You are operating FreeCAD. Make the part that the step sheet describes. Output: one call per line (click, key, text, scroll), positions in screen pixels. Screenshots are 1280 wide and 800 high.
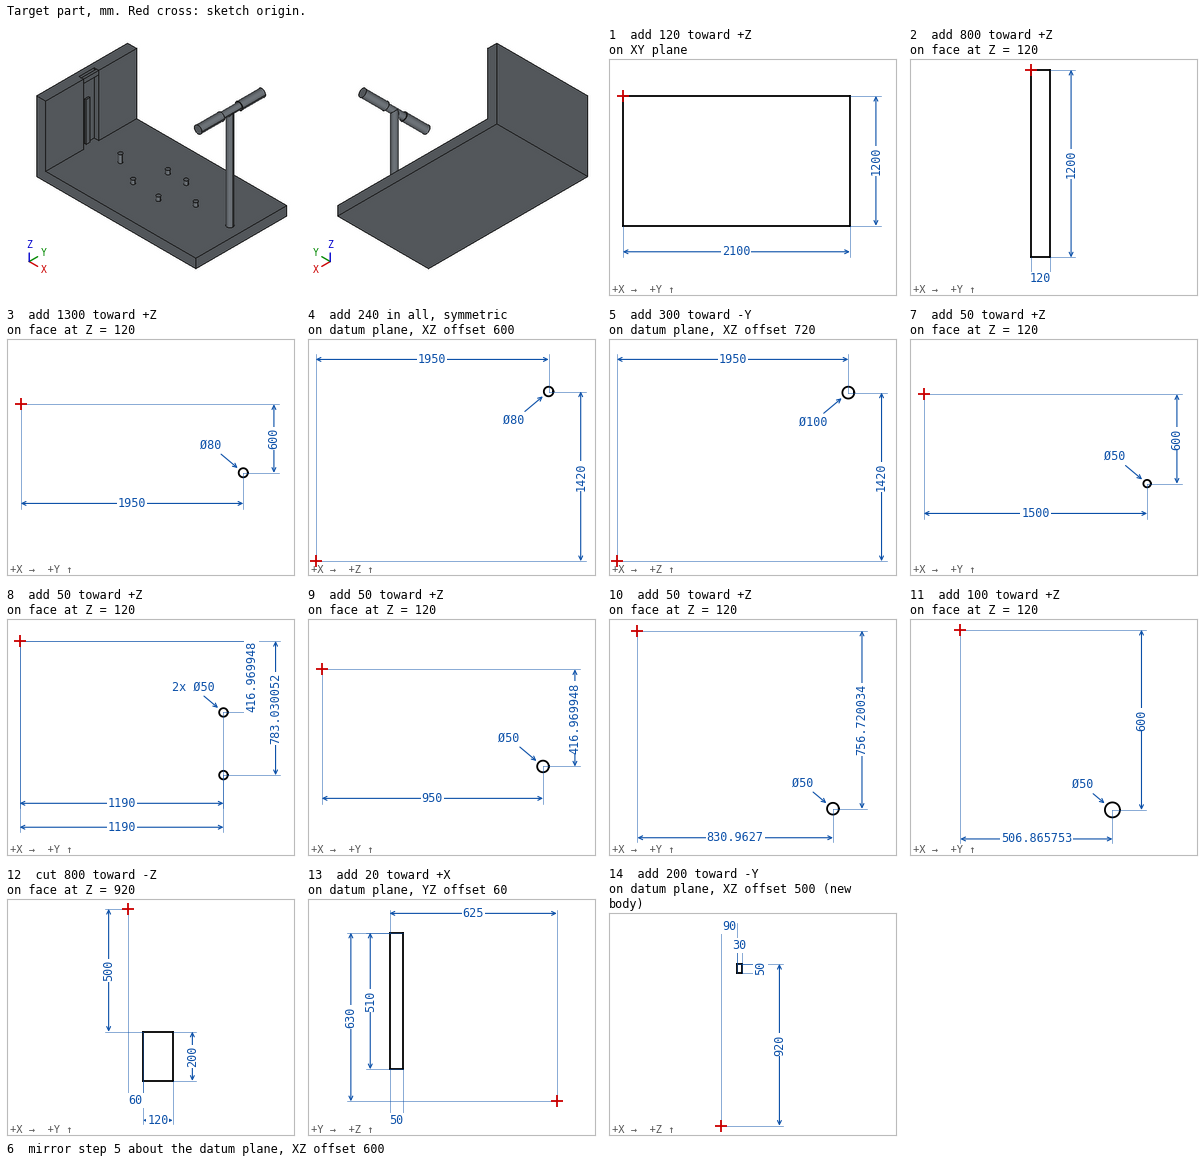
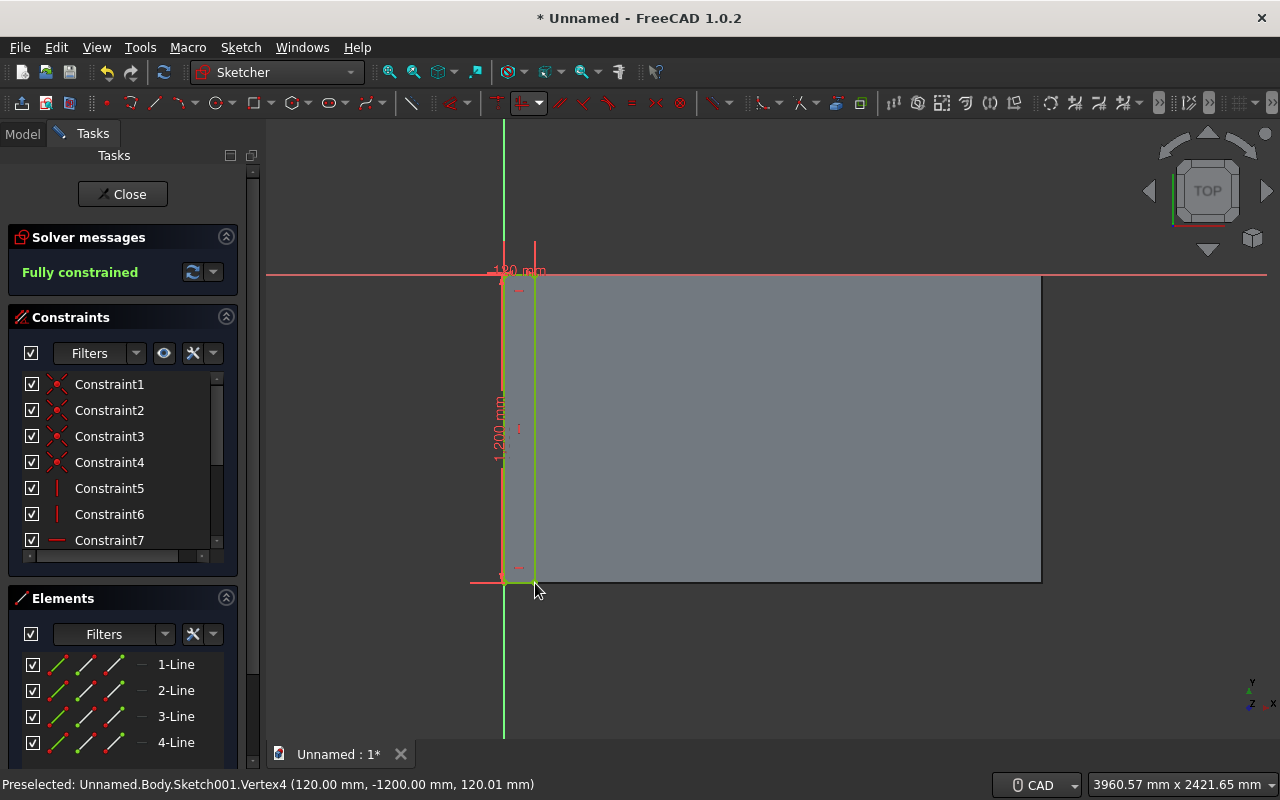
click(123, 194)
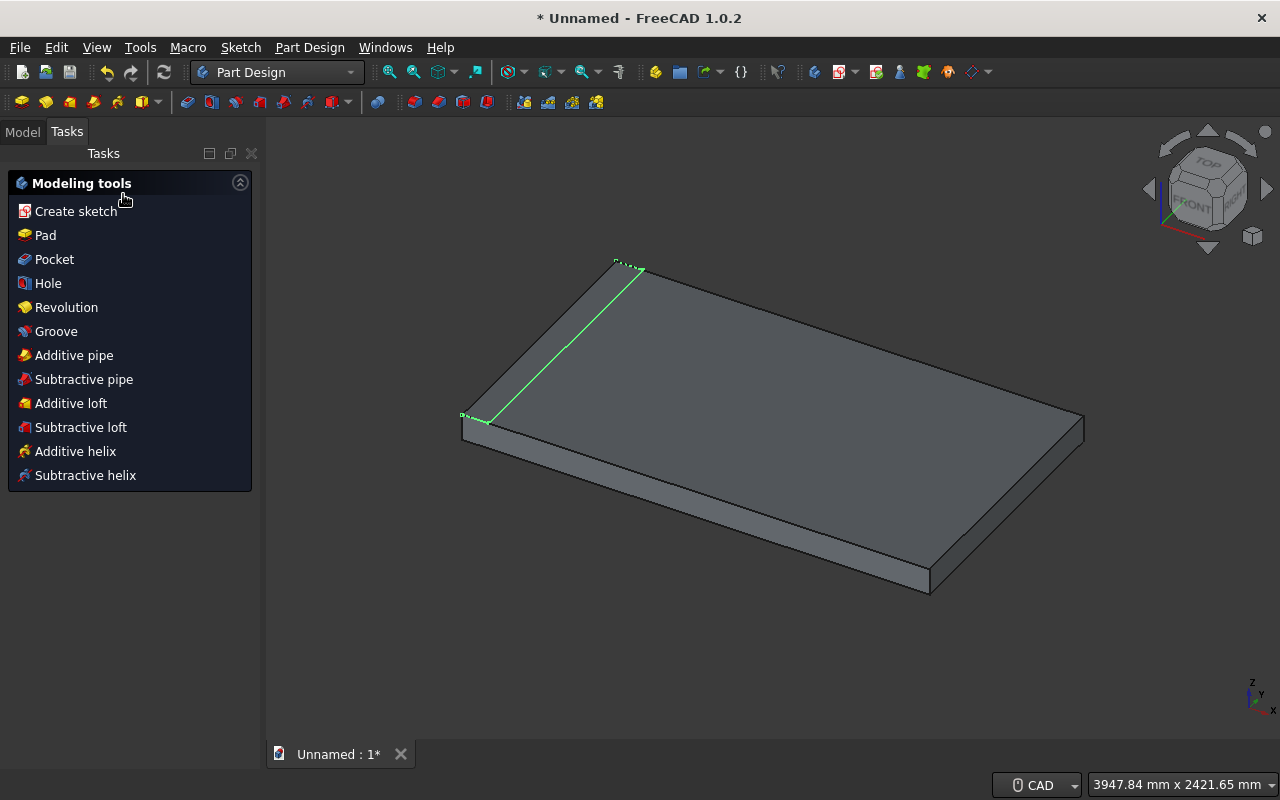
click(22, 102)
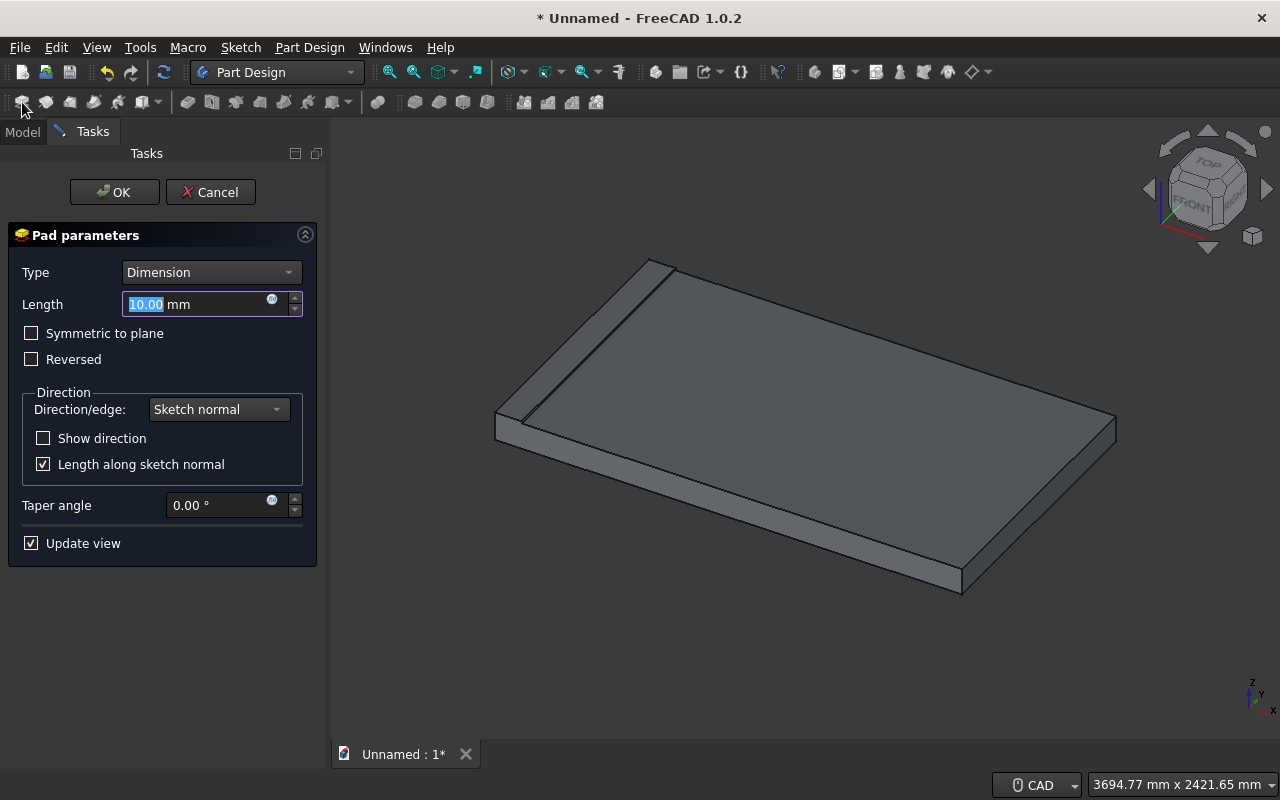
text(800)
key(Tab)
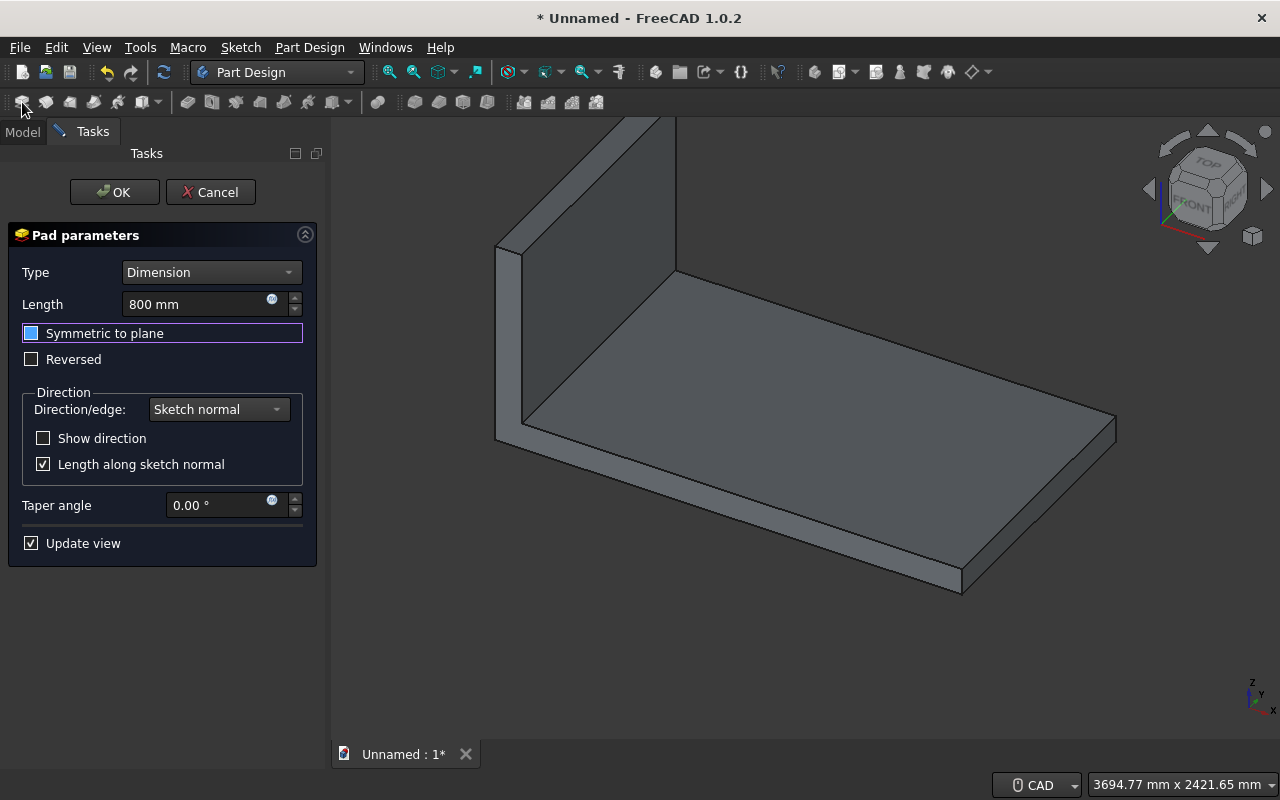
click(115, 192)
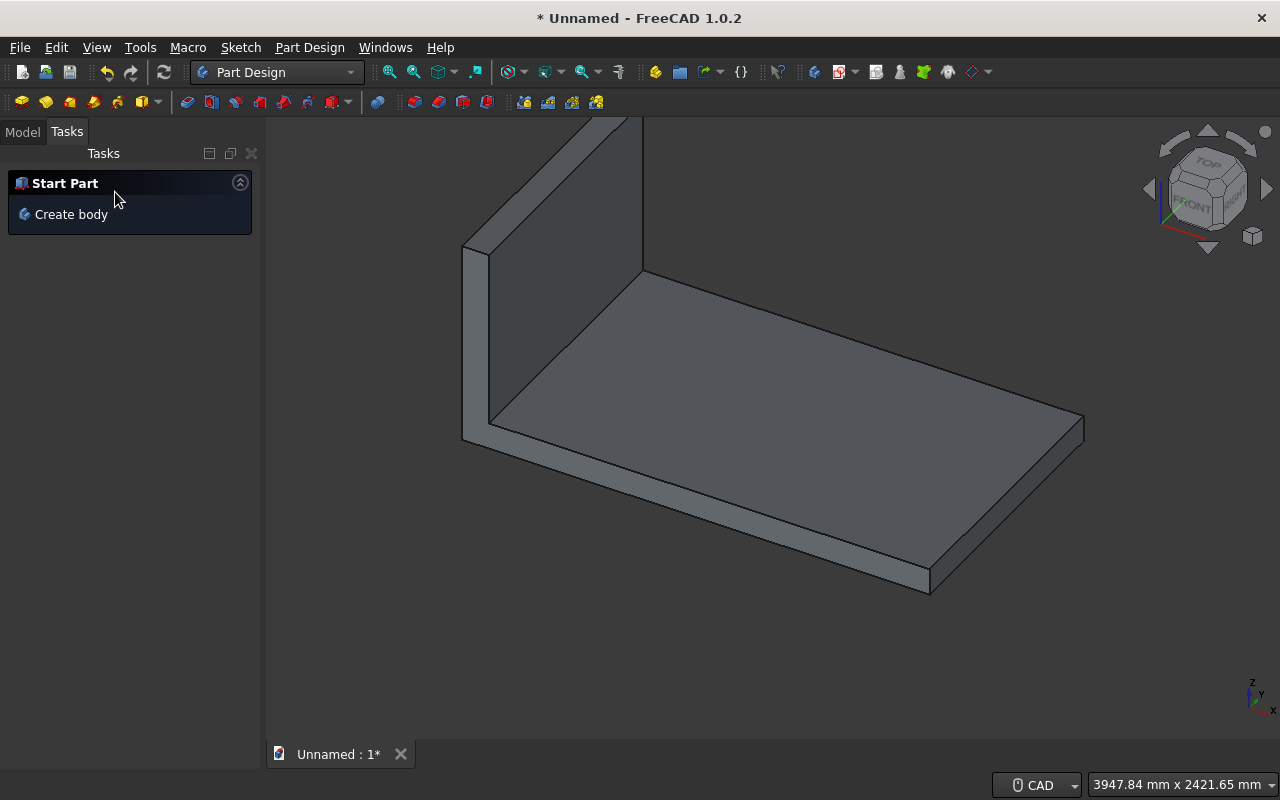
key(v)
key(f)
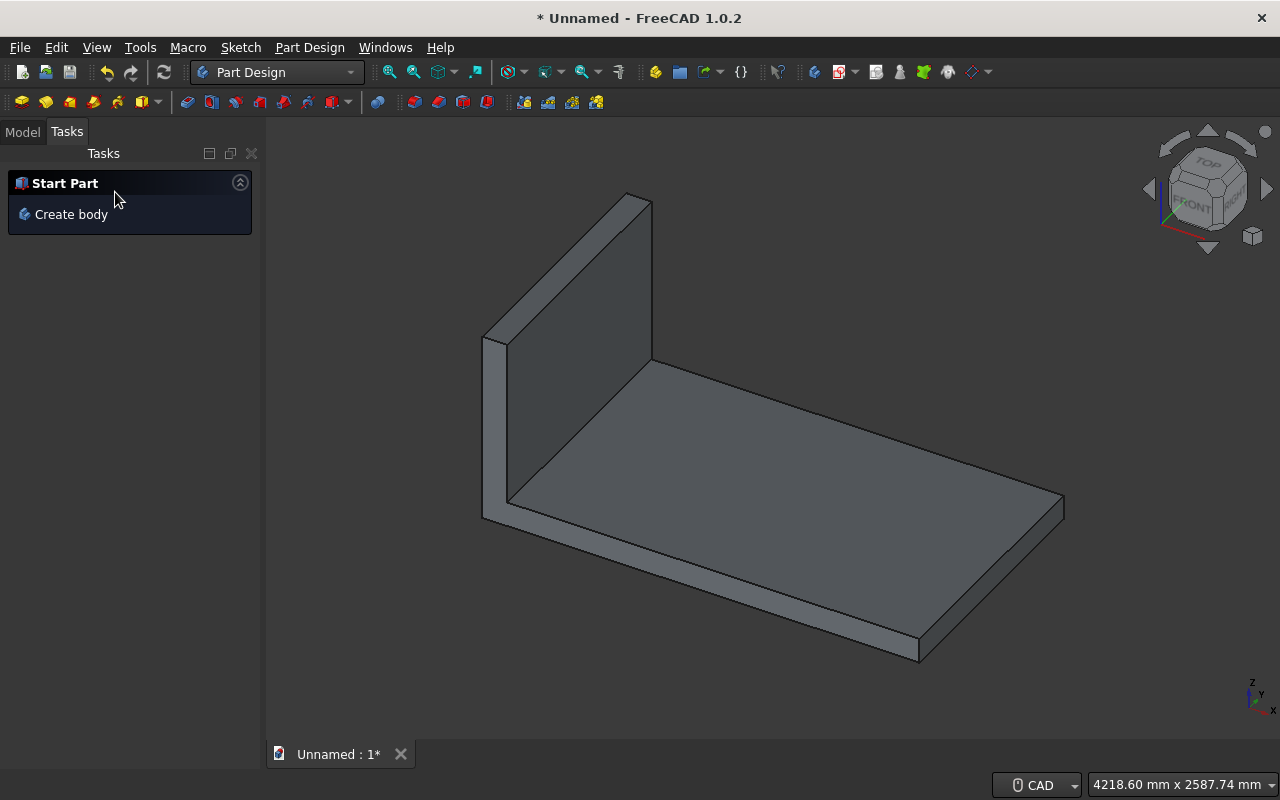
click(844, 518)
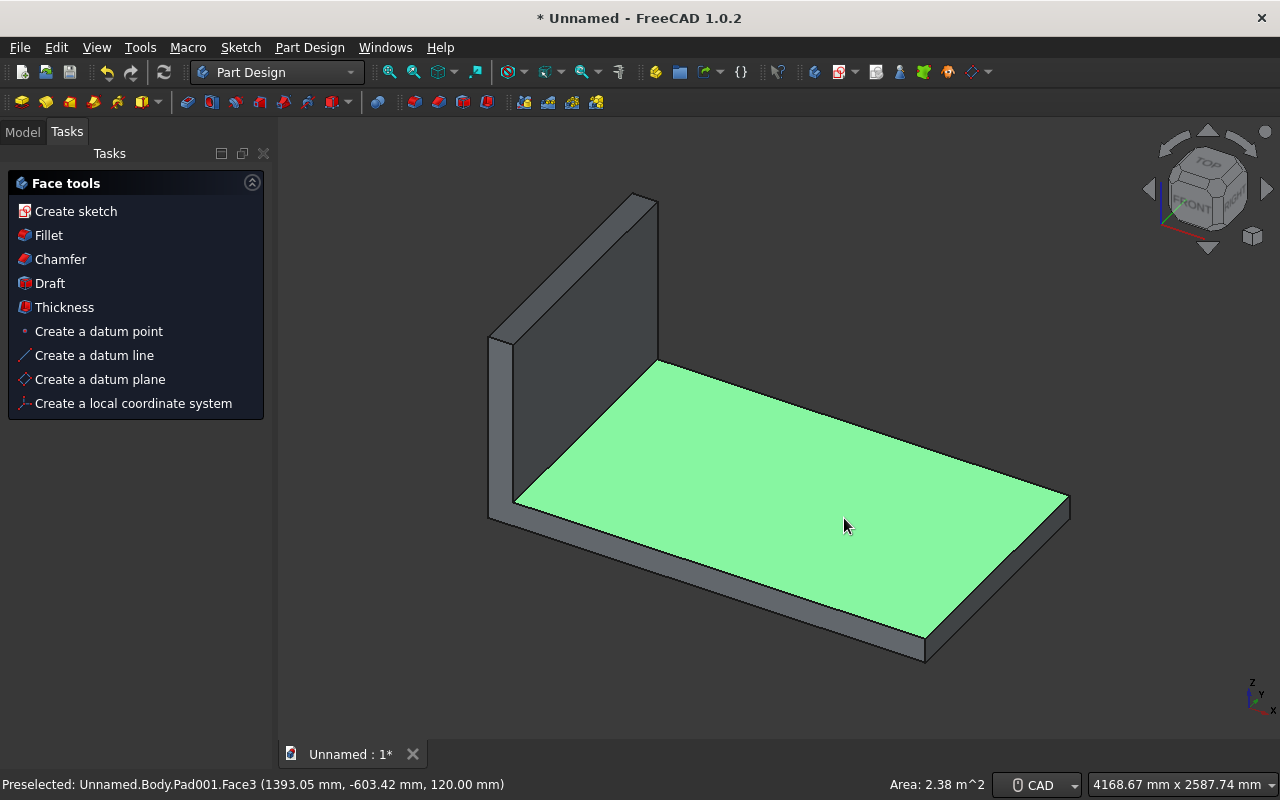
click(840, 72)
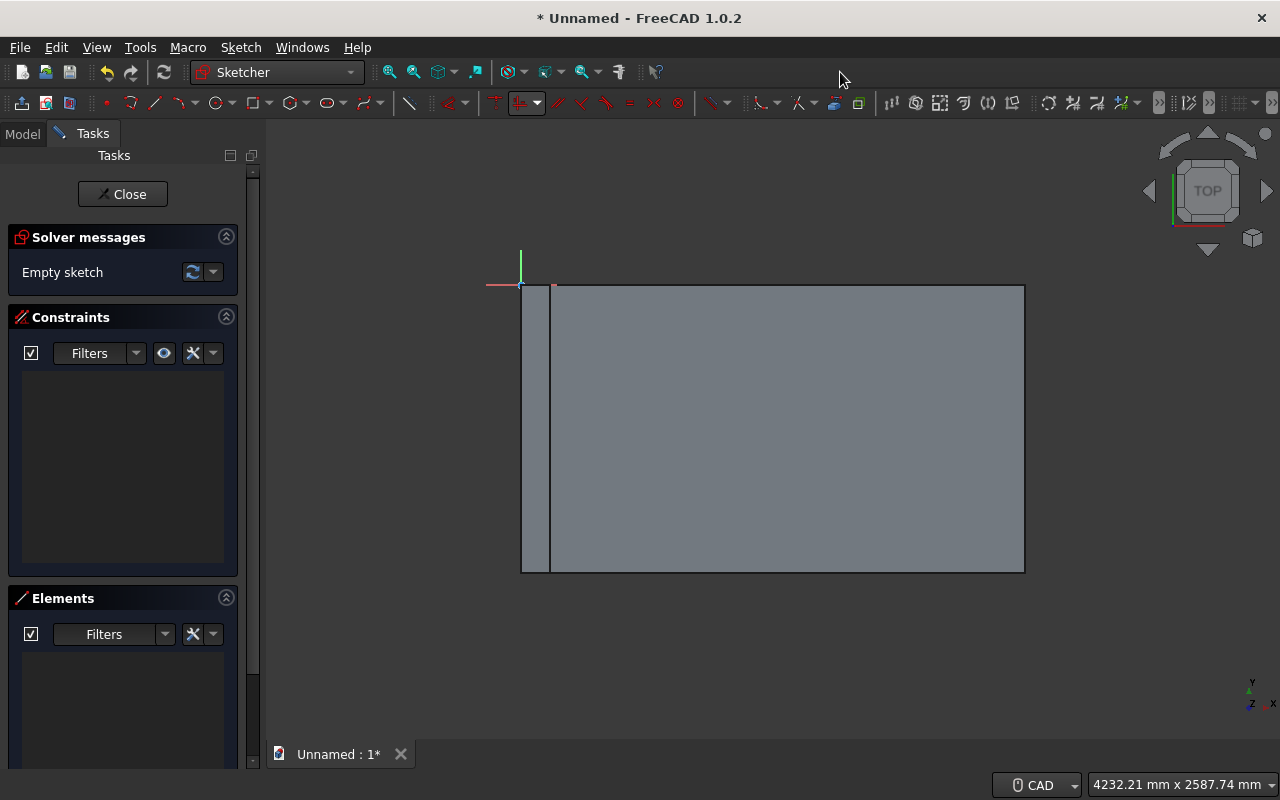
scroll(1004, 429, up, 15)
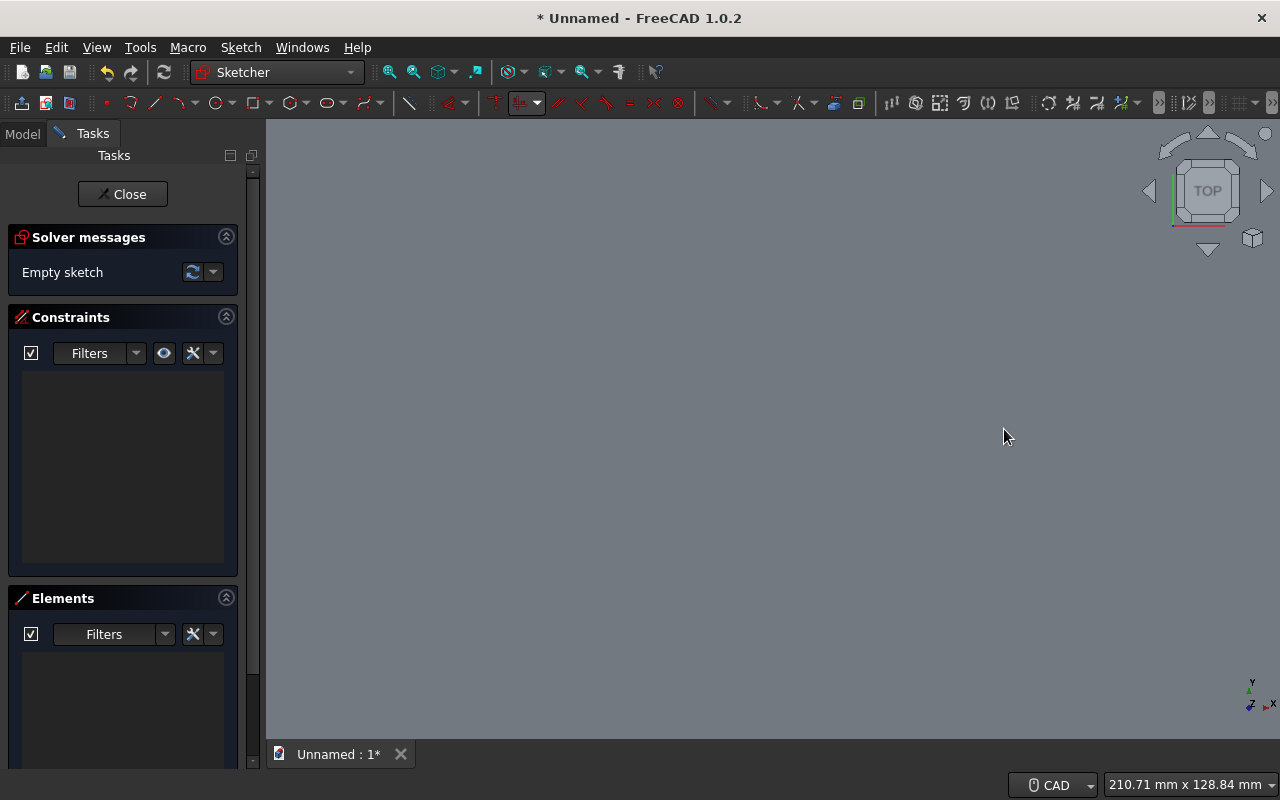
click(216, 104)